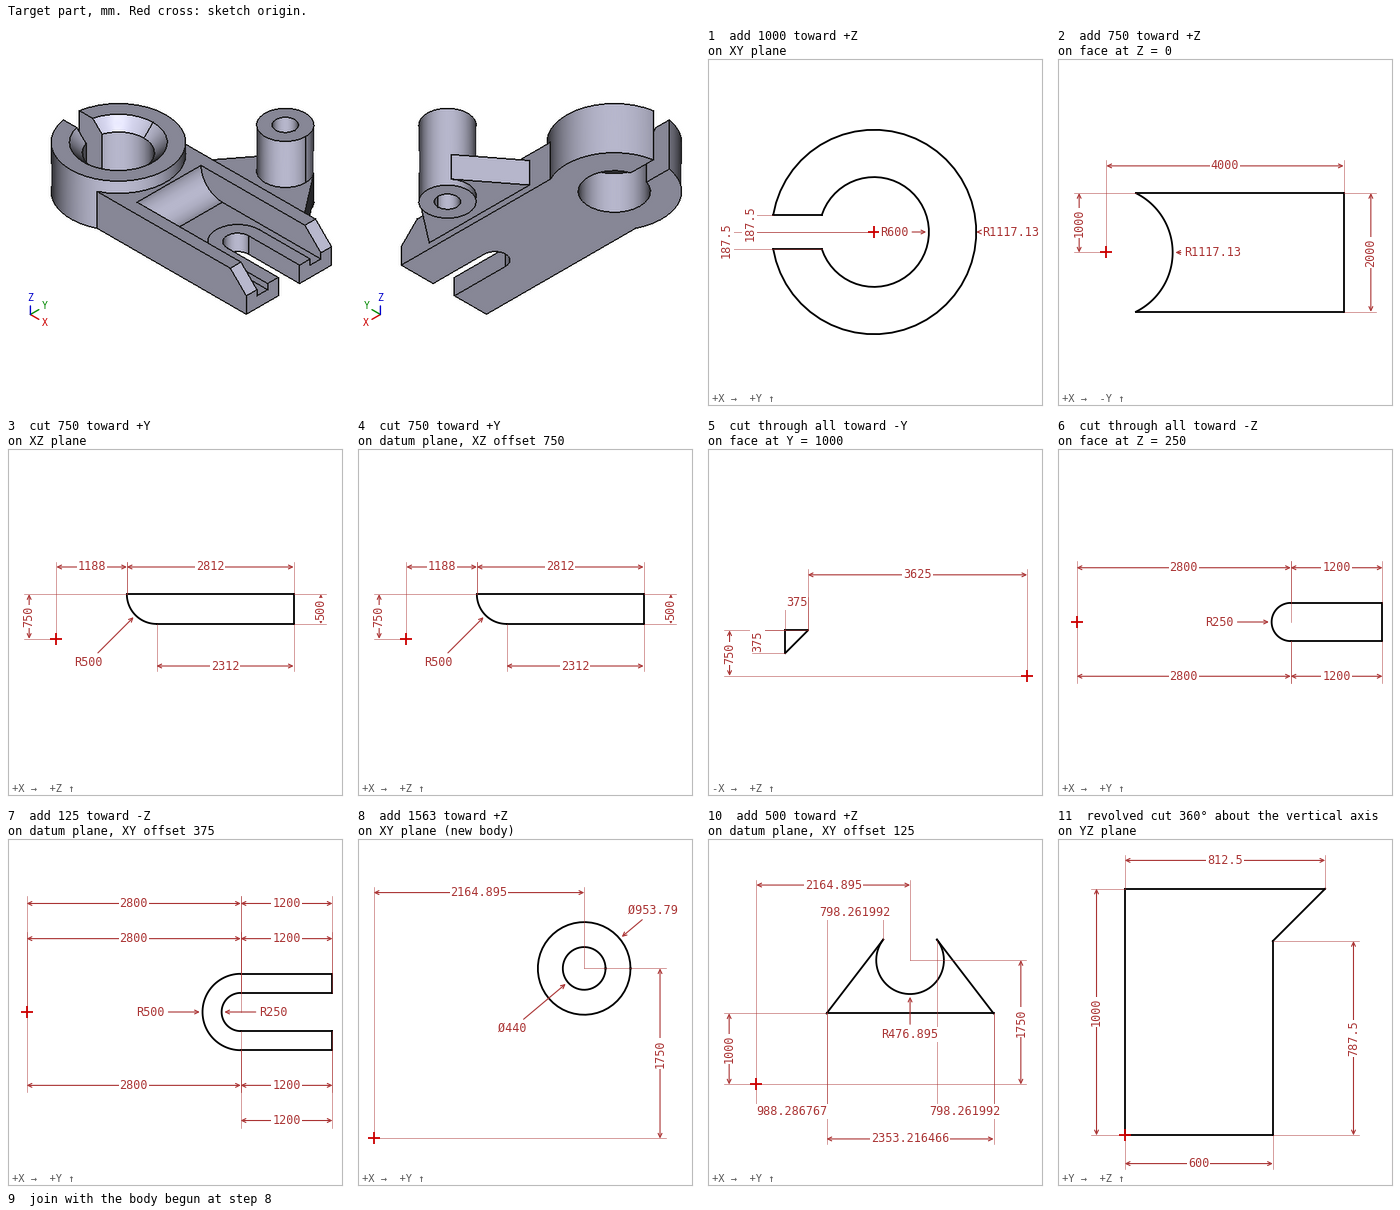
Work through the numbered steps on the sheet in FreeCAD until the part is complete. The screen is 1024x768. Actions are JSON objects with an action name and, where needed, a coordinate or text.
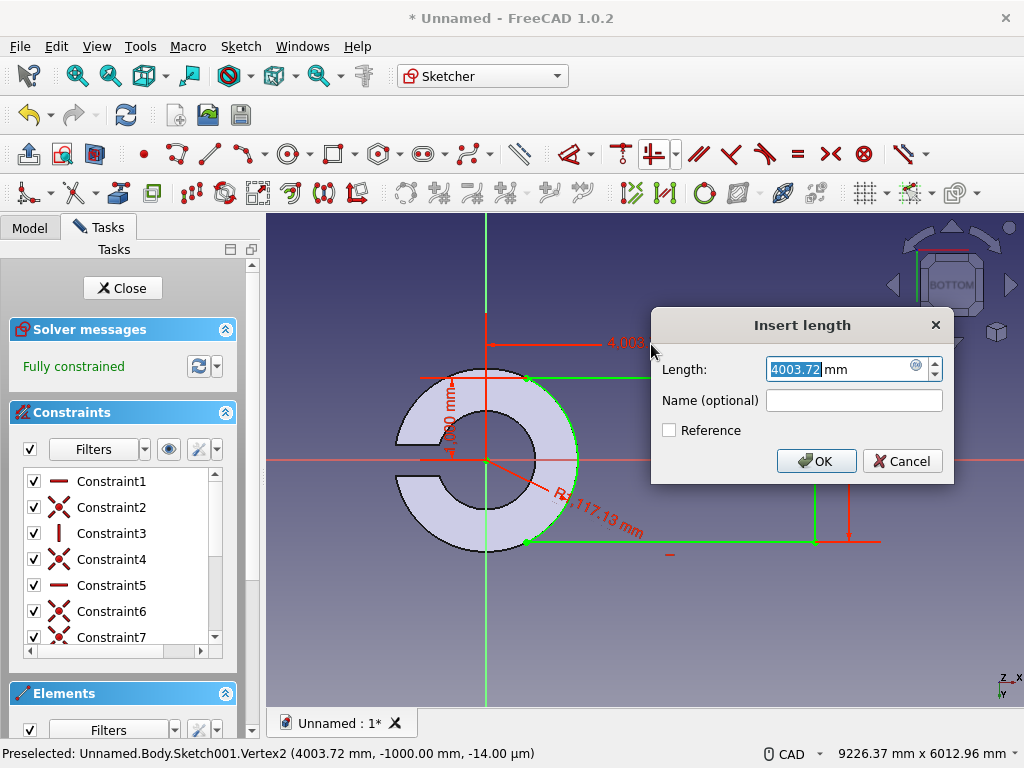
{"action": "type", "text": "4000"}
{"action": "key", "text": "Return"}
{"action": "key", "text": "Escape"}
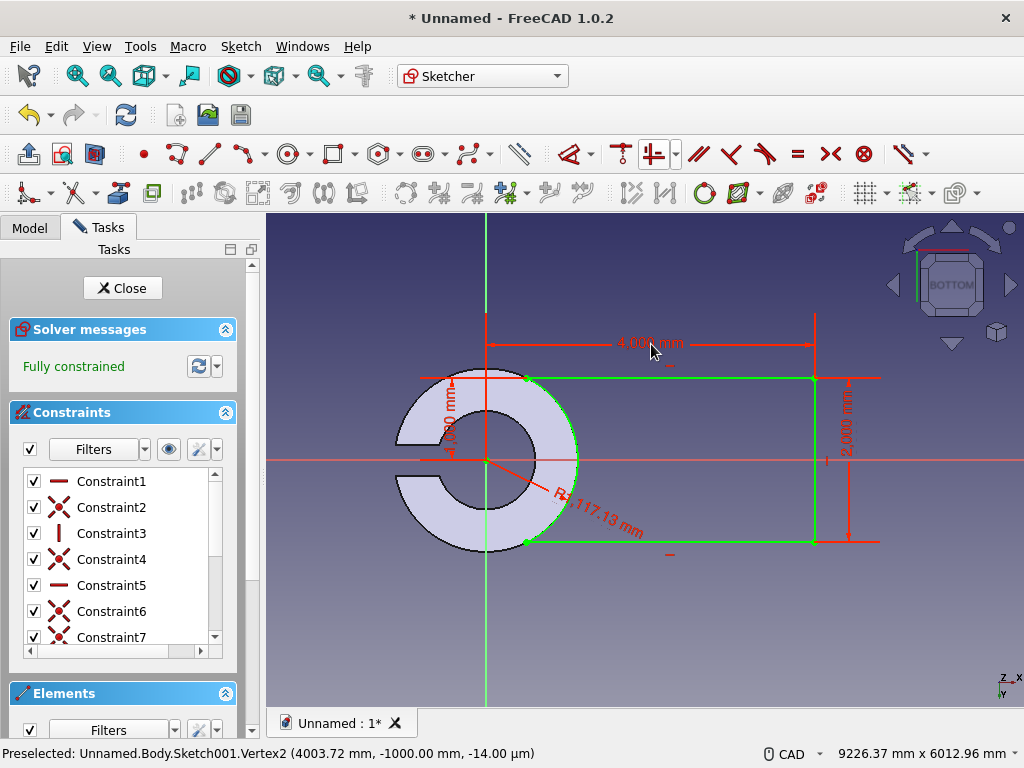
{"action": "left_click", "coordinate": [123, 288]}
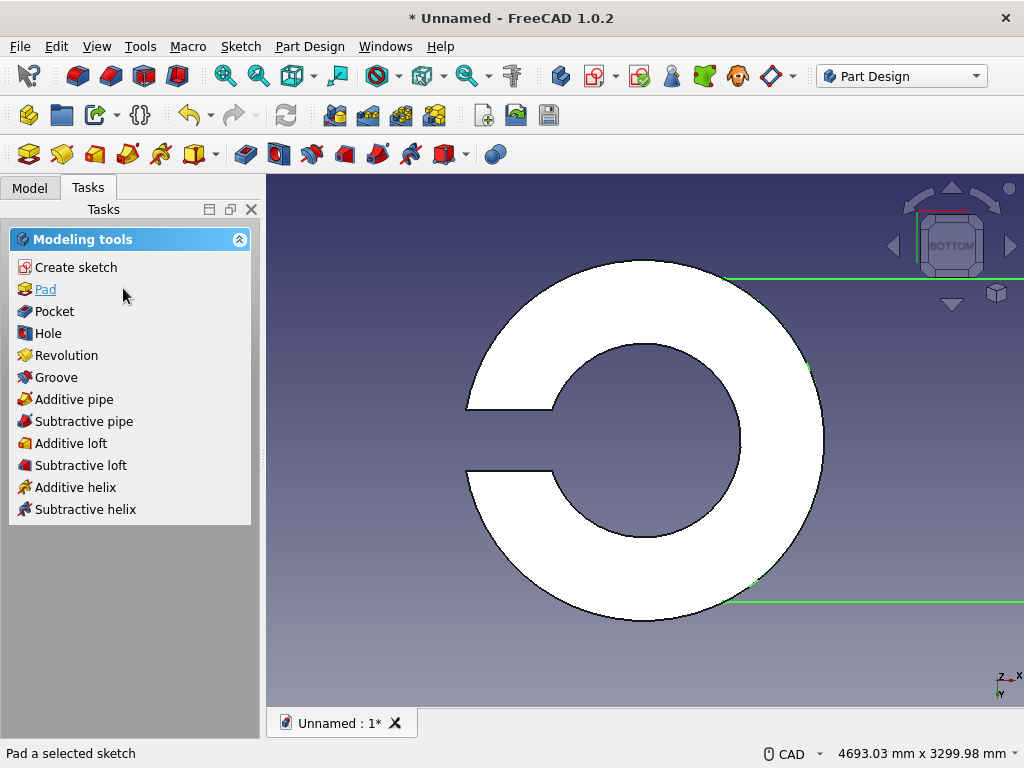
{"action": "left_click", "coordinate": [29, 154]}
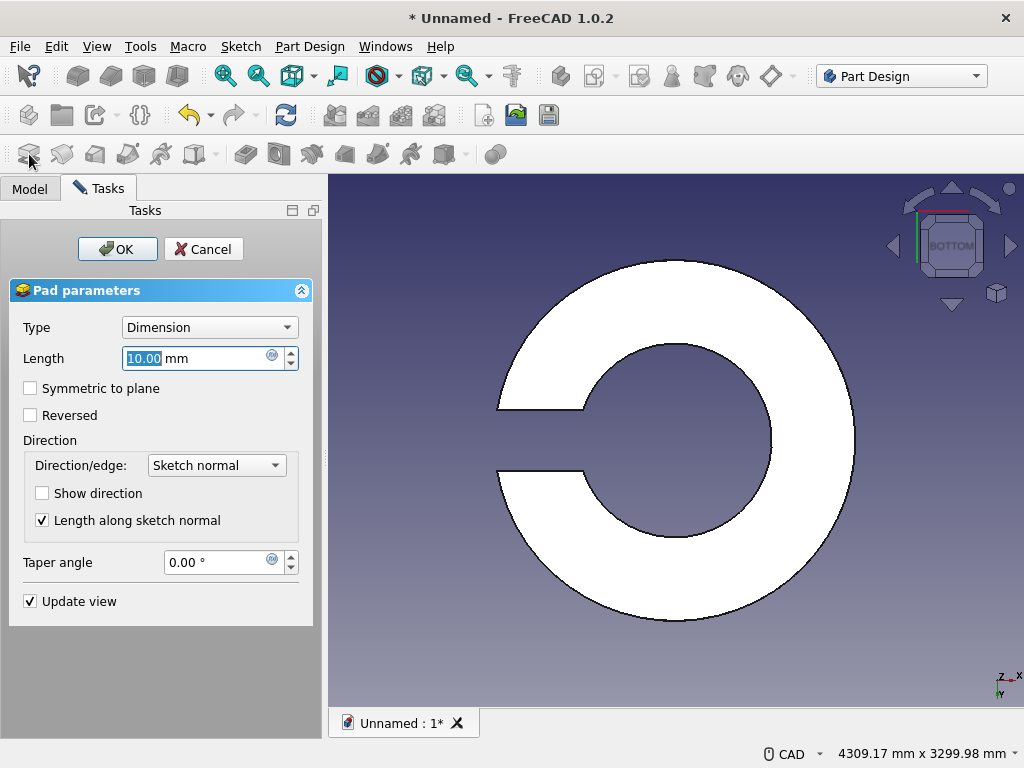
{"action": "type", "text": "750"}
{"action": "key", "text": "Tab"}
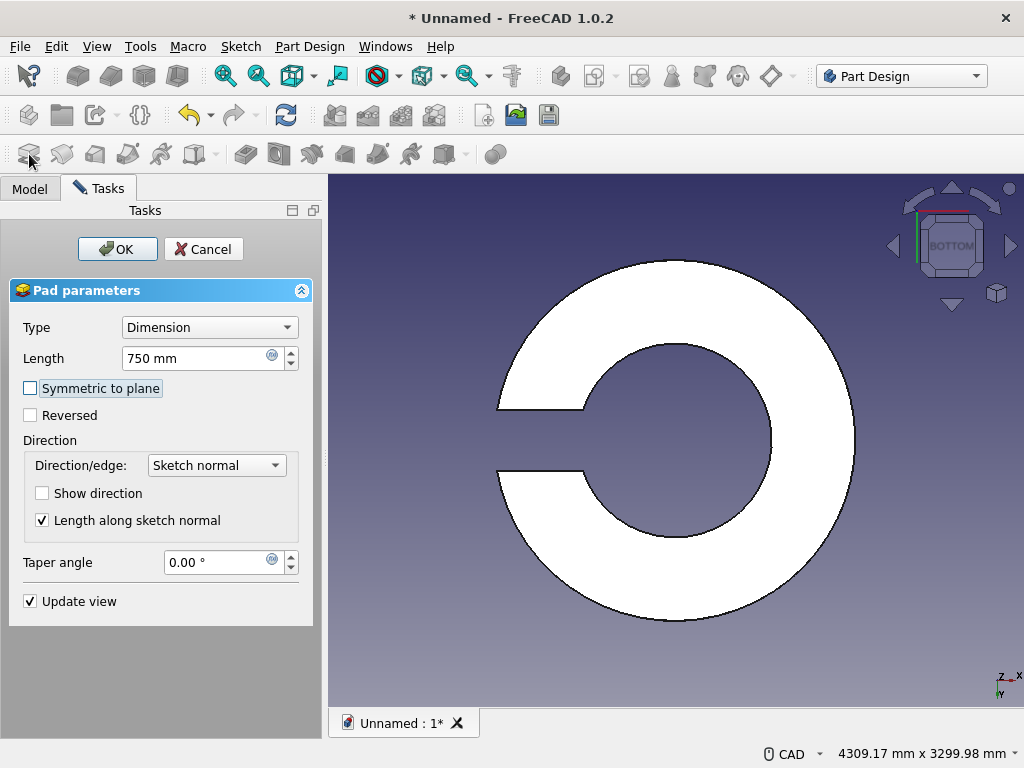
{"action": "left_click", "coordinate": [31, 415]}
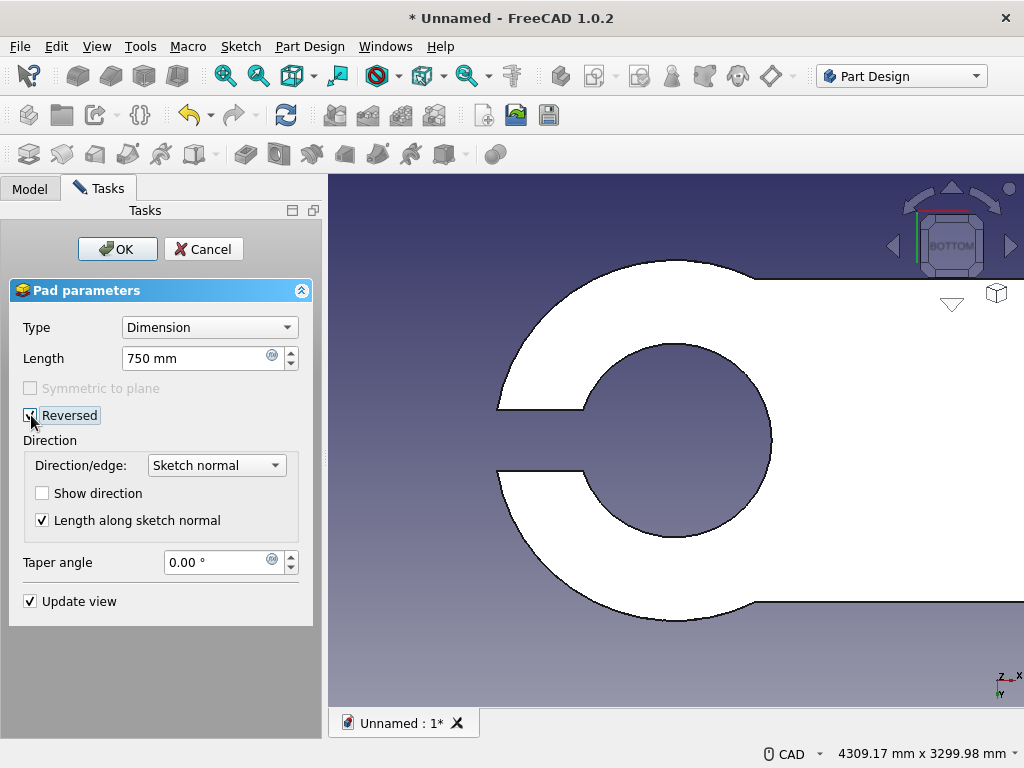
{"action": "left_click", "coordinate": [118, 249]}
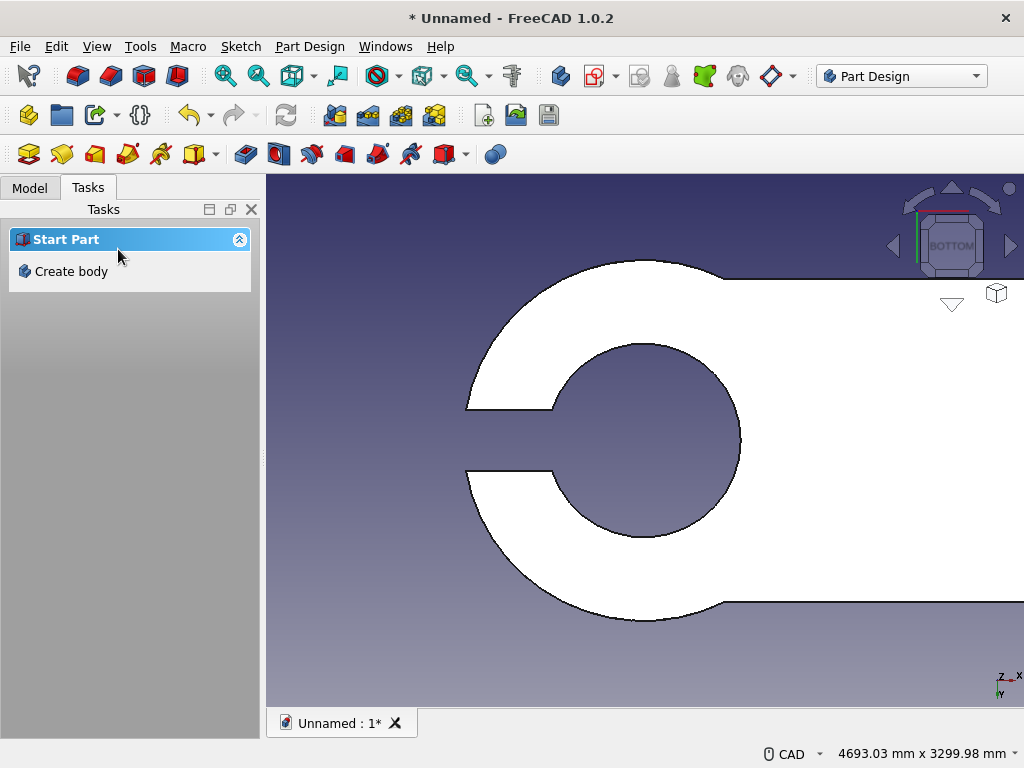
{"action": "key", "text": "v f"}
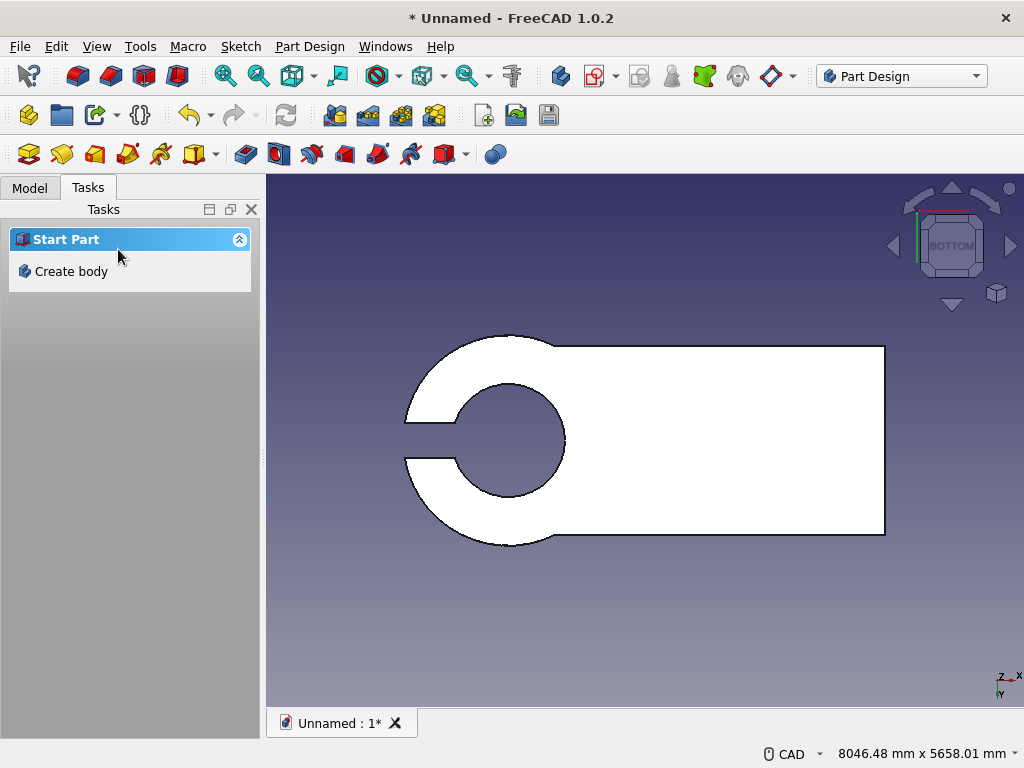
{"action": "left_click", "coordinate": [594, 76]}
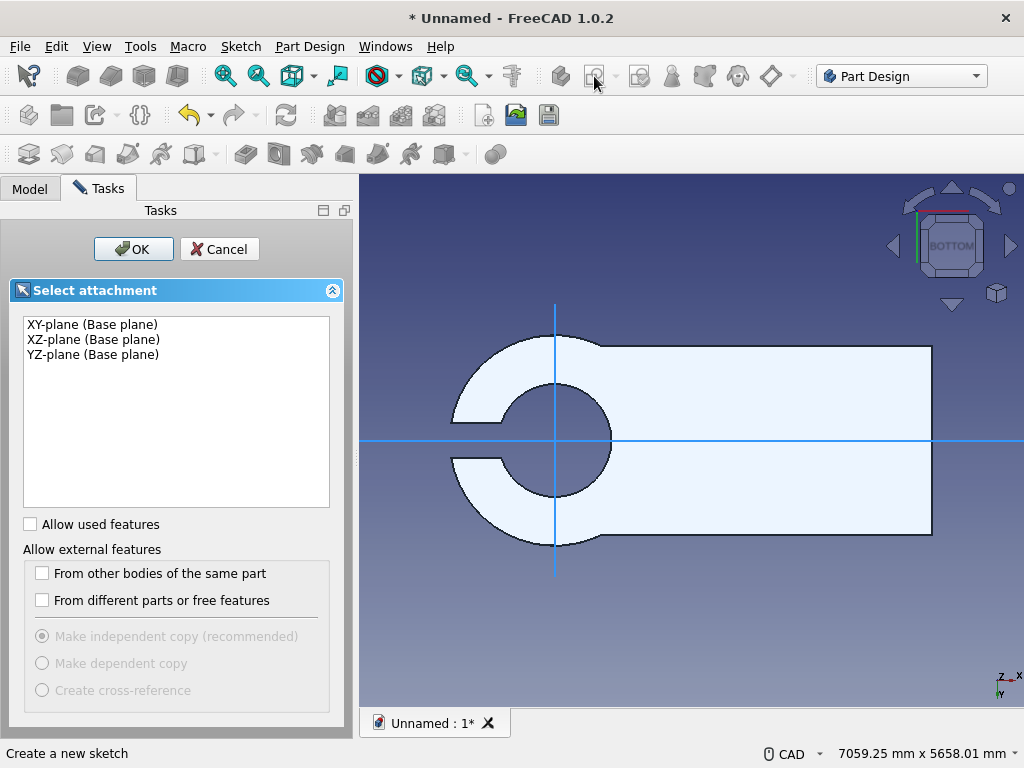
{"action": "left_click", "coordinate": [84, 340]}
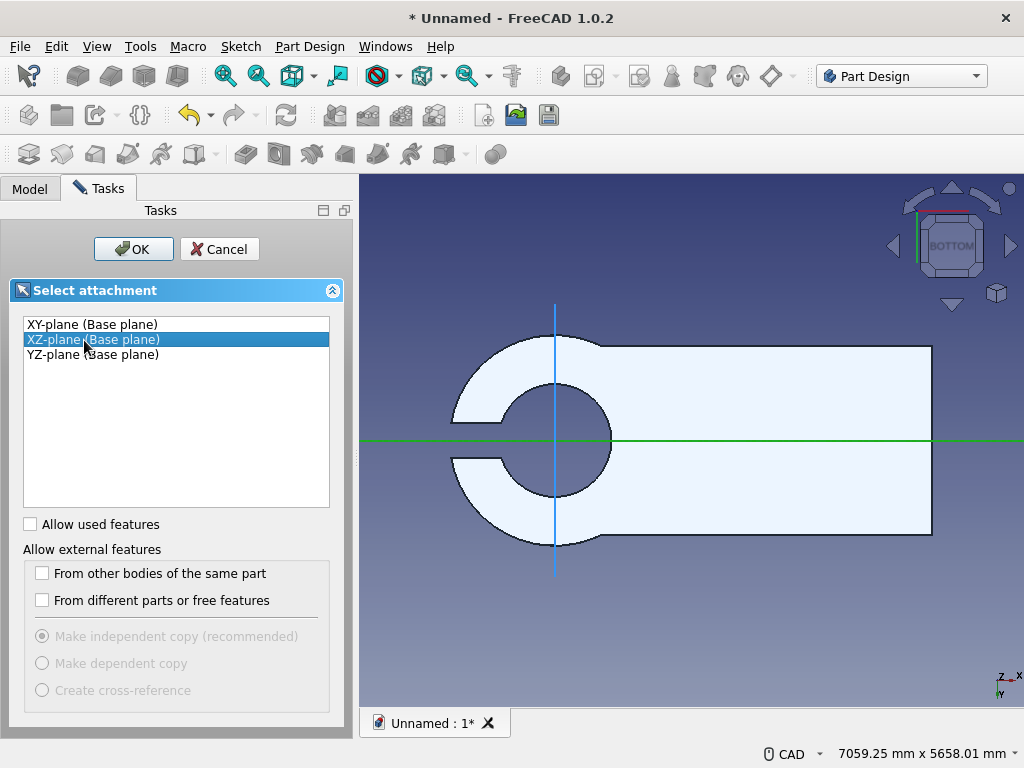
{"action": "left_click", "coordinate": [134, 249]}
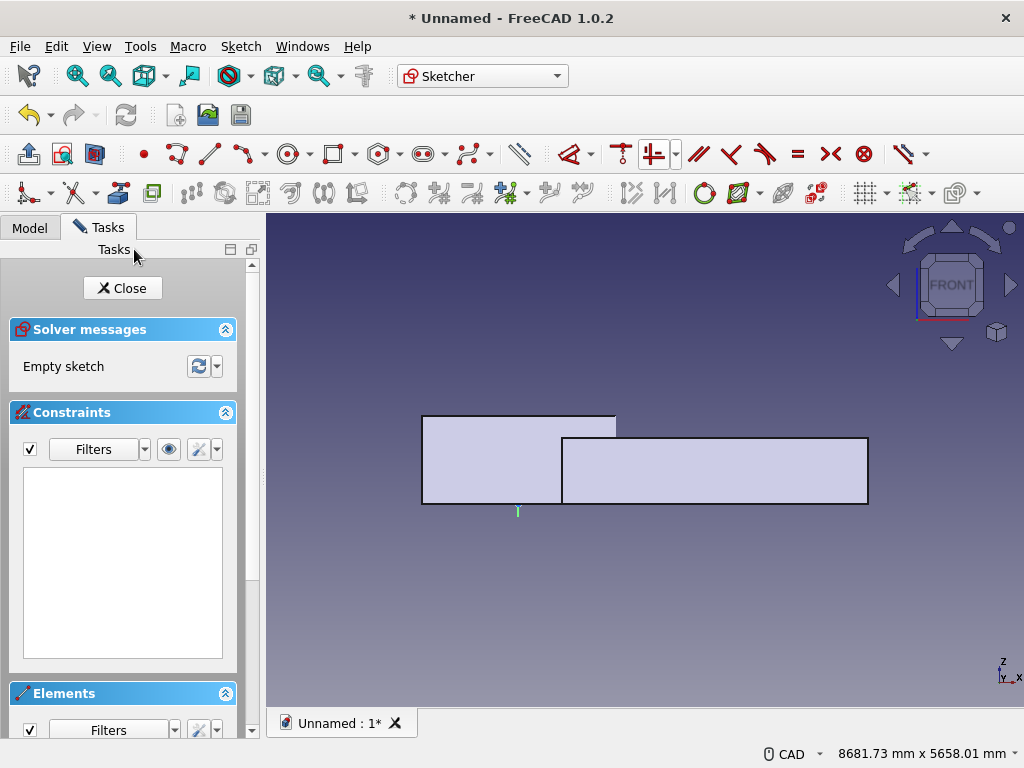
{"action": "key", "text": "q s"}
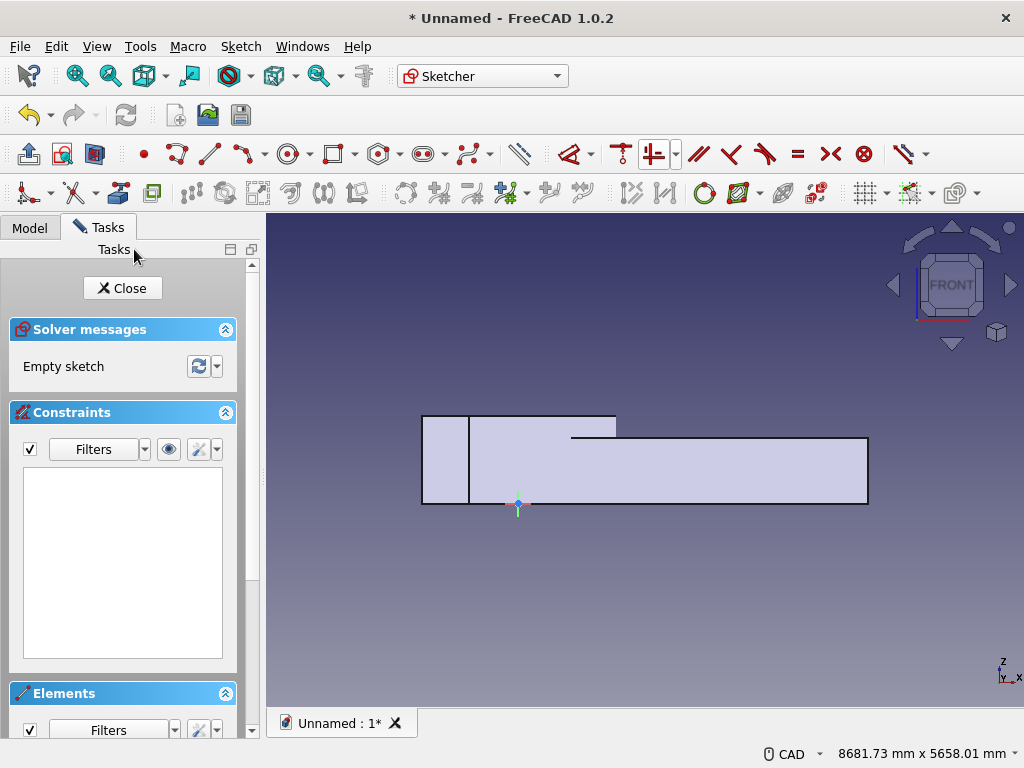
{"action": "scroll", "coordinate": [294, 411], "scroll_direction": "down", "scroll_amount": 1}